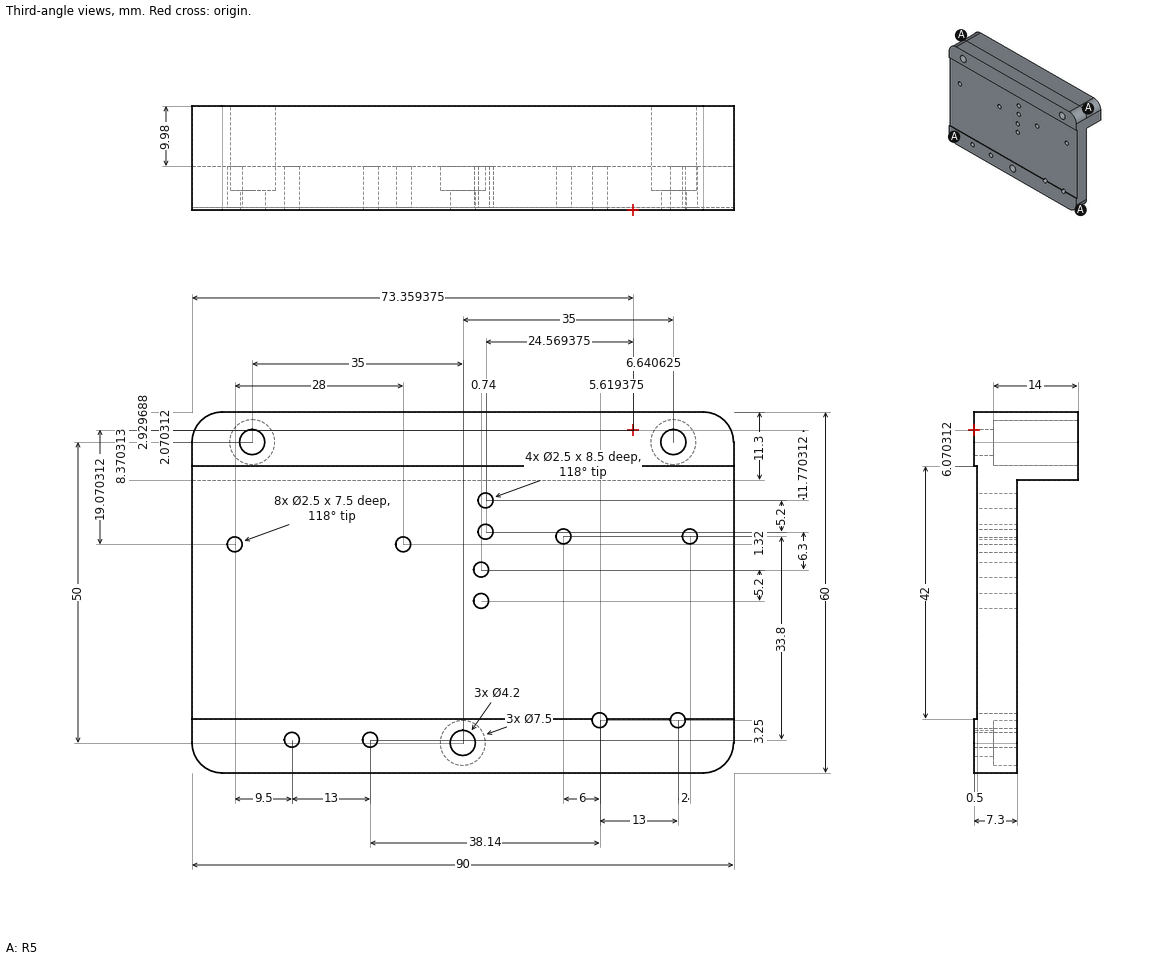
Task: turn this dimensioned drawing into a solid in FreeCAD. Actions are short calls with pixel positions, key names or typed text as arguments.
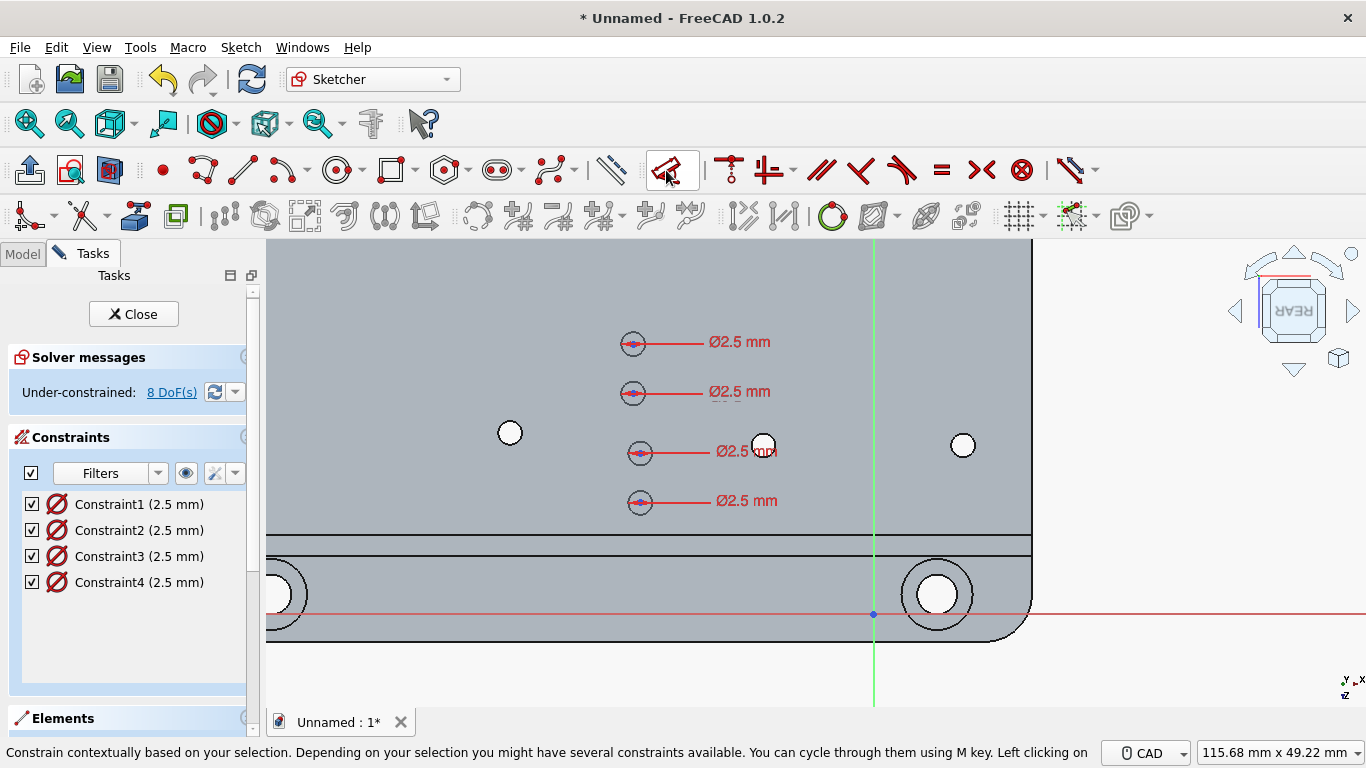
click(640, 503)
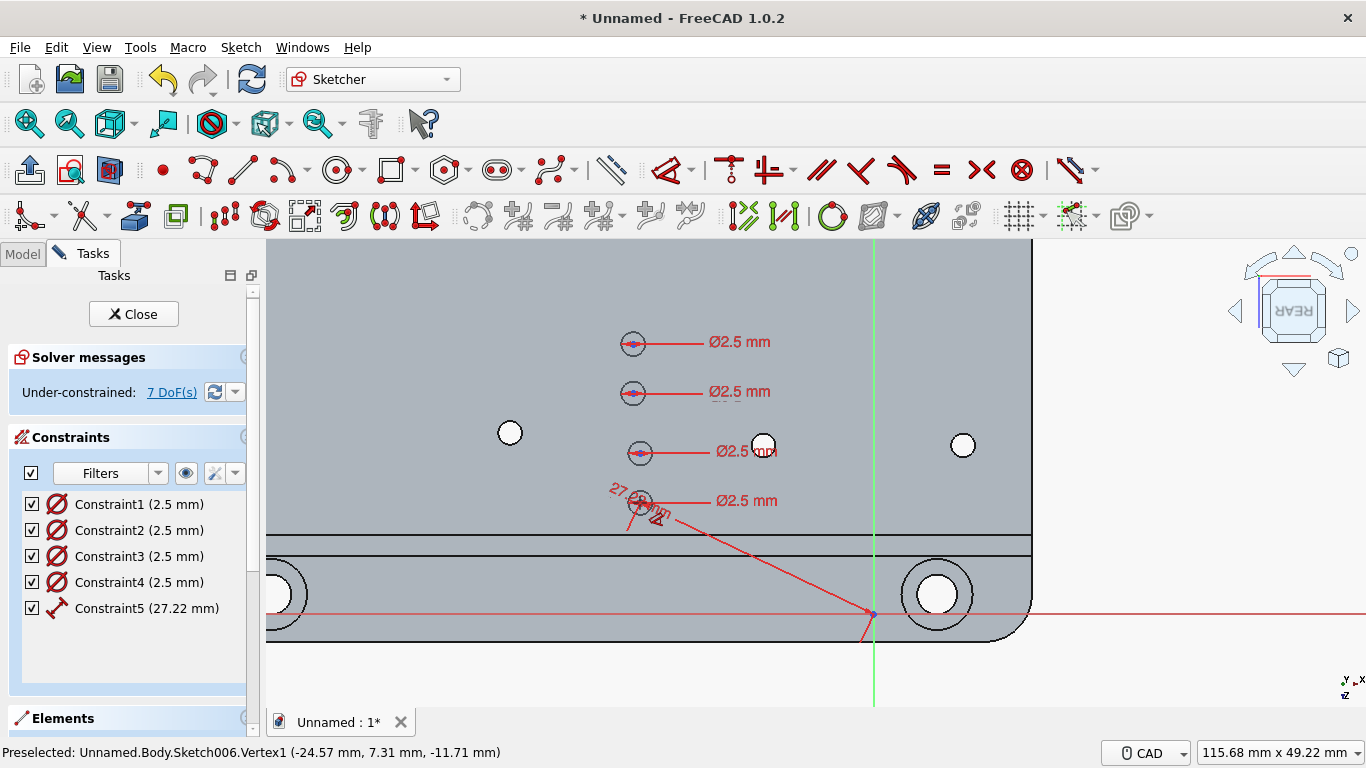
click(640, 453)
click(606, 478)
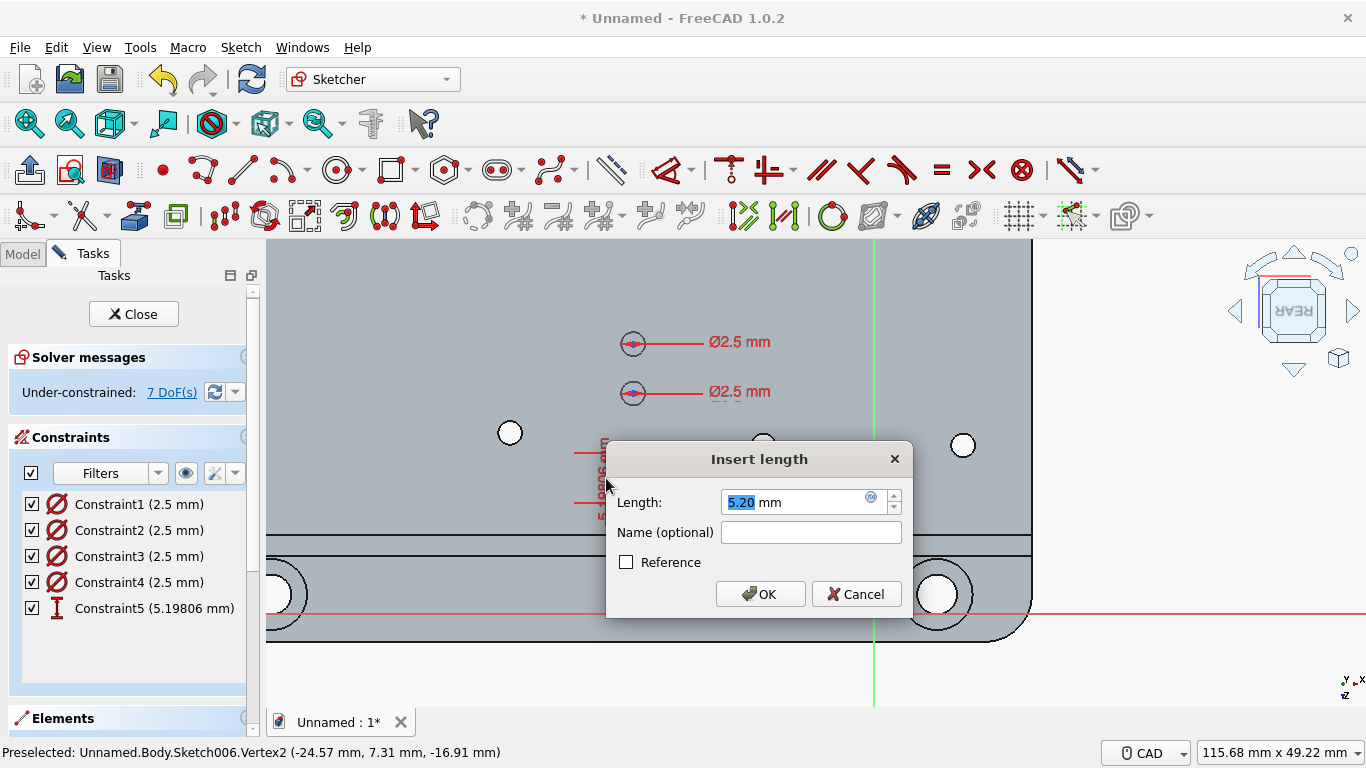
text(5.2)
key(Return)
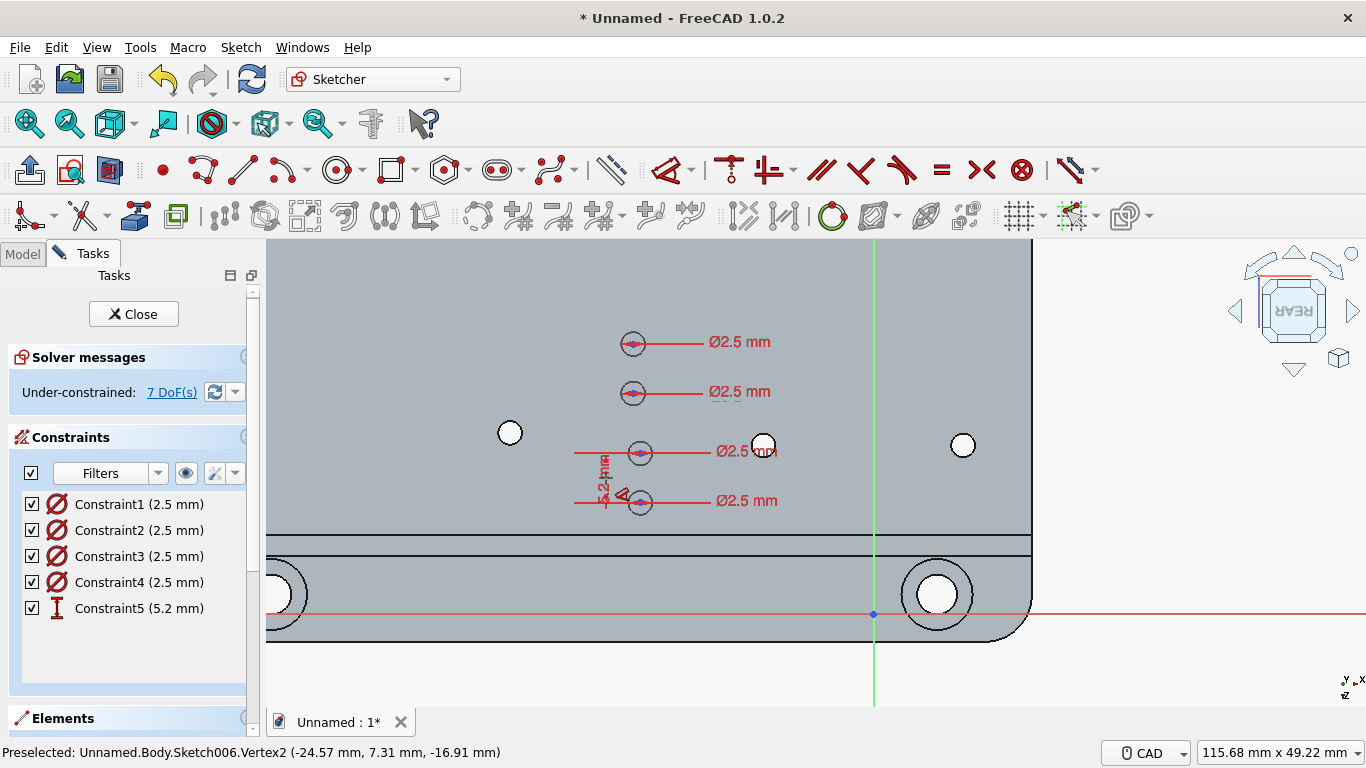
click(640, 453)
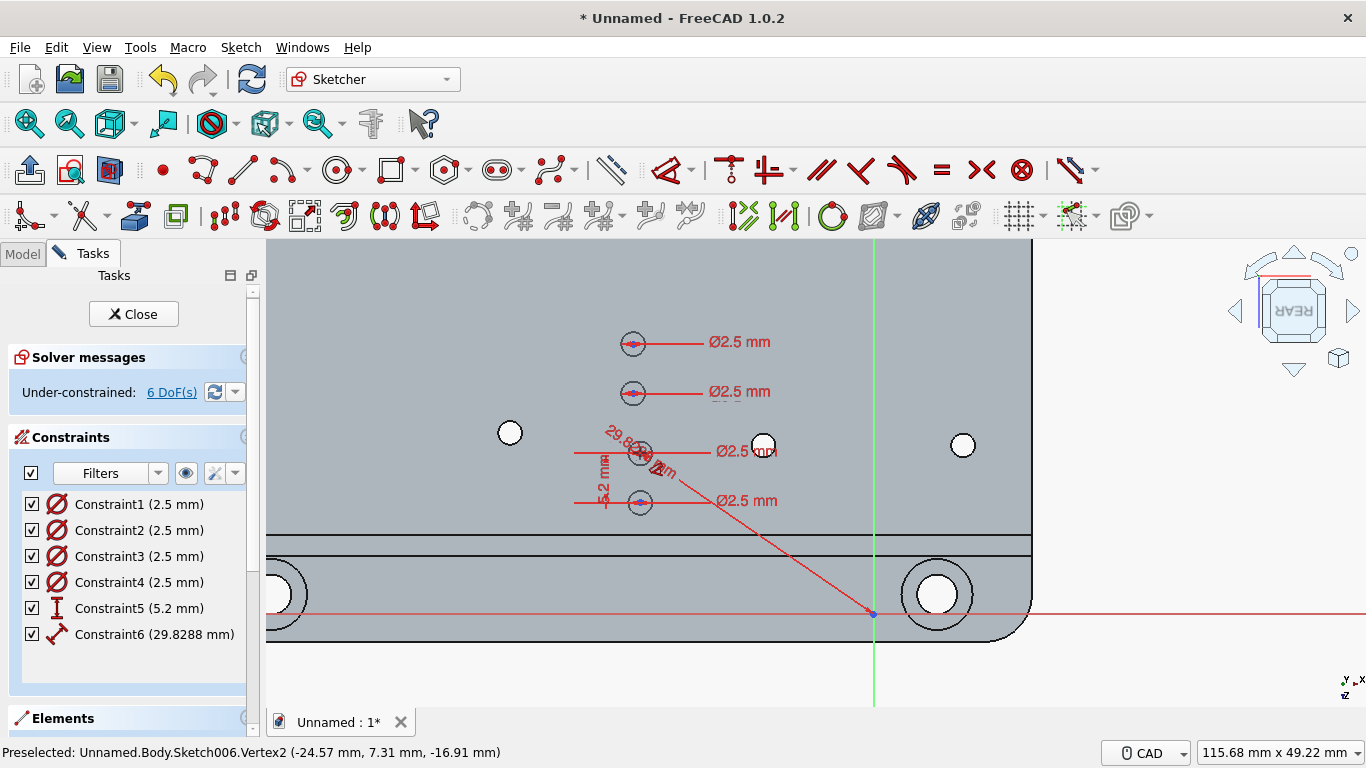
click(633, 394)
click(599, 423)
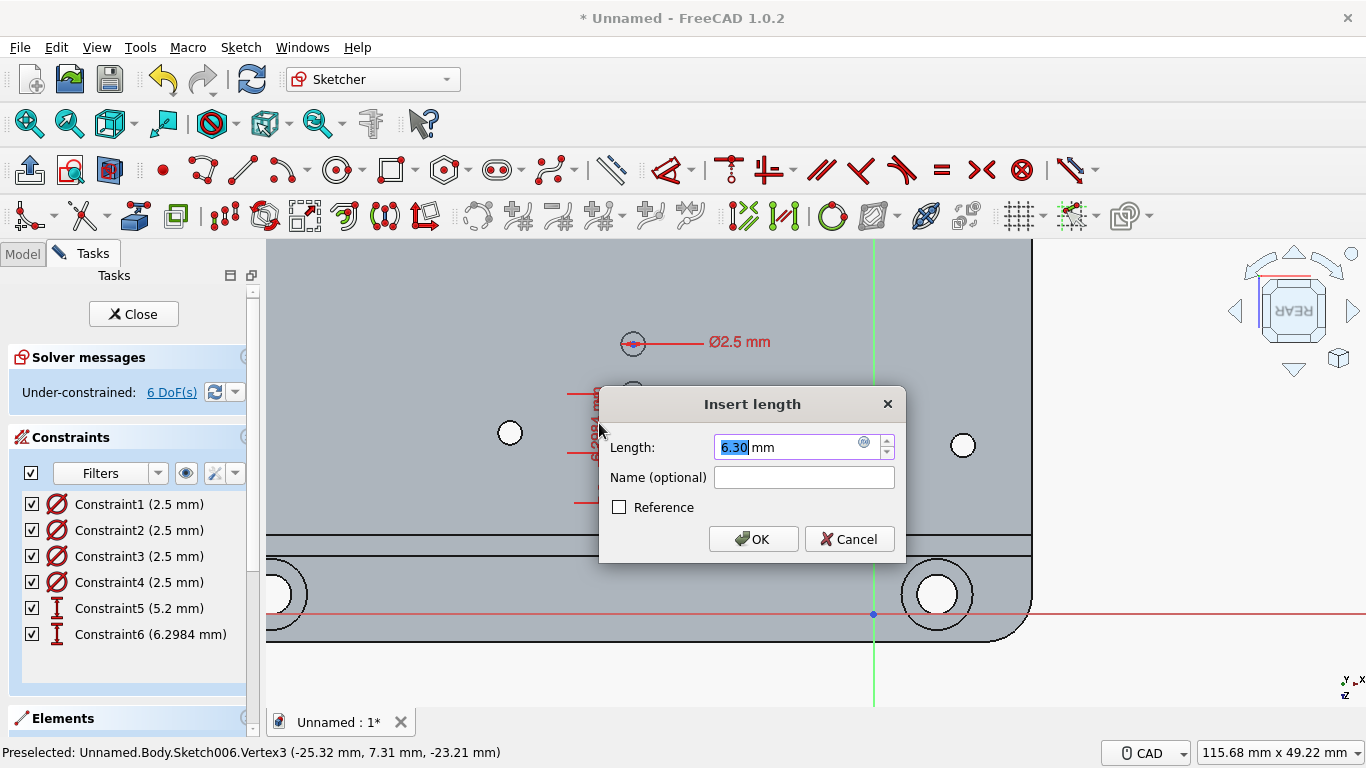
text(6.3)
key(Return)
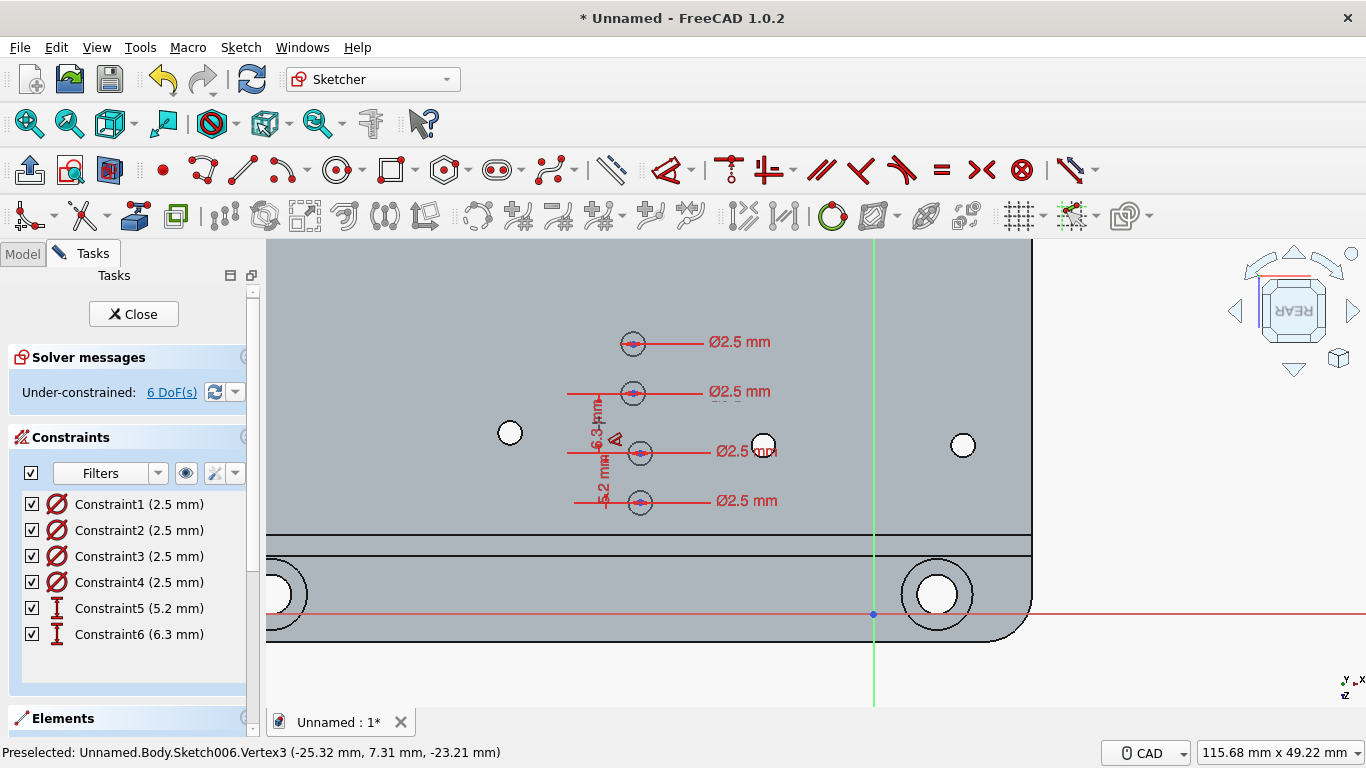
click(633, 394)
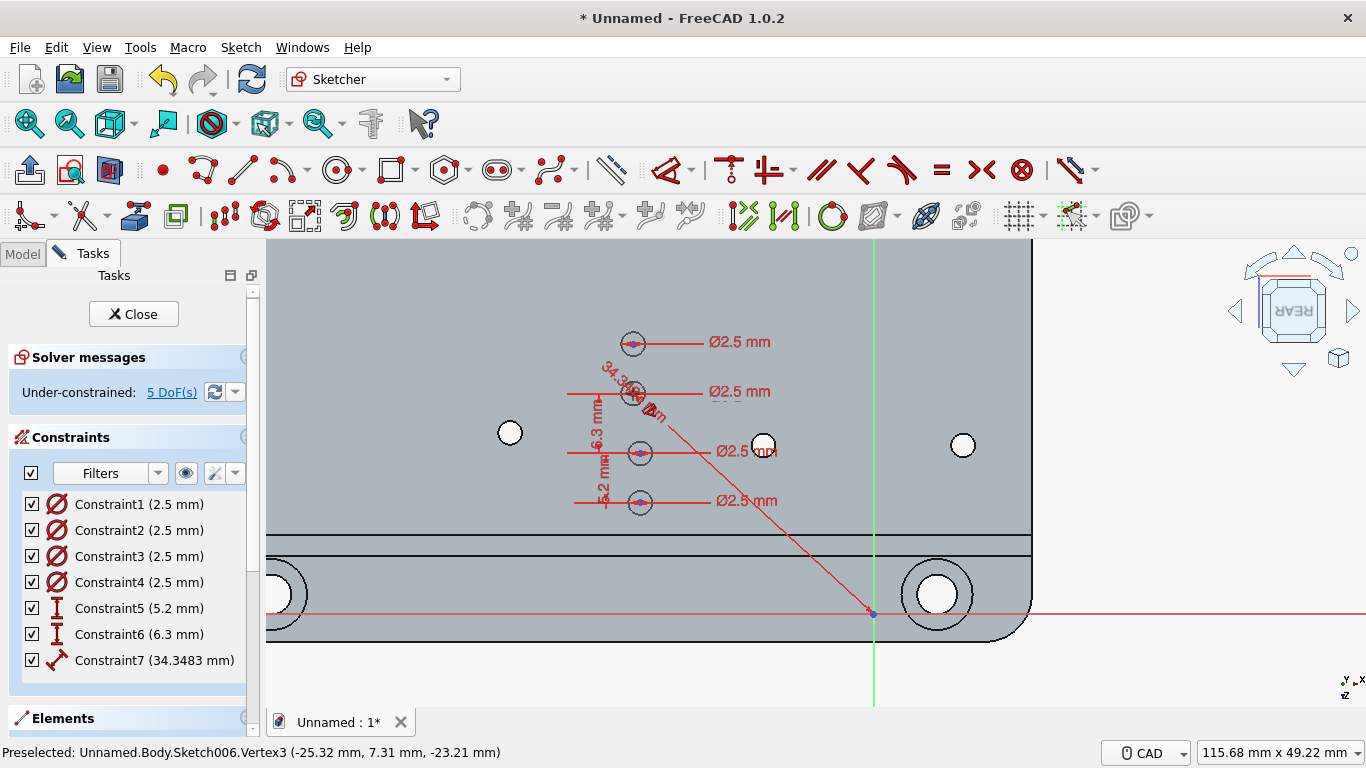
click(633, 344)
click(599, 369)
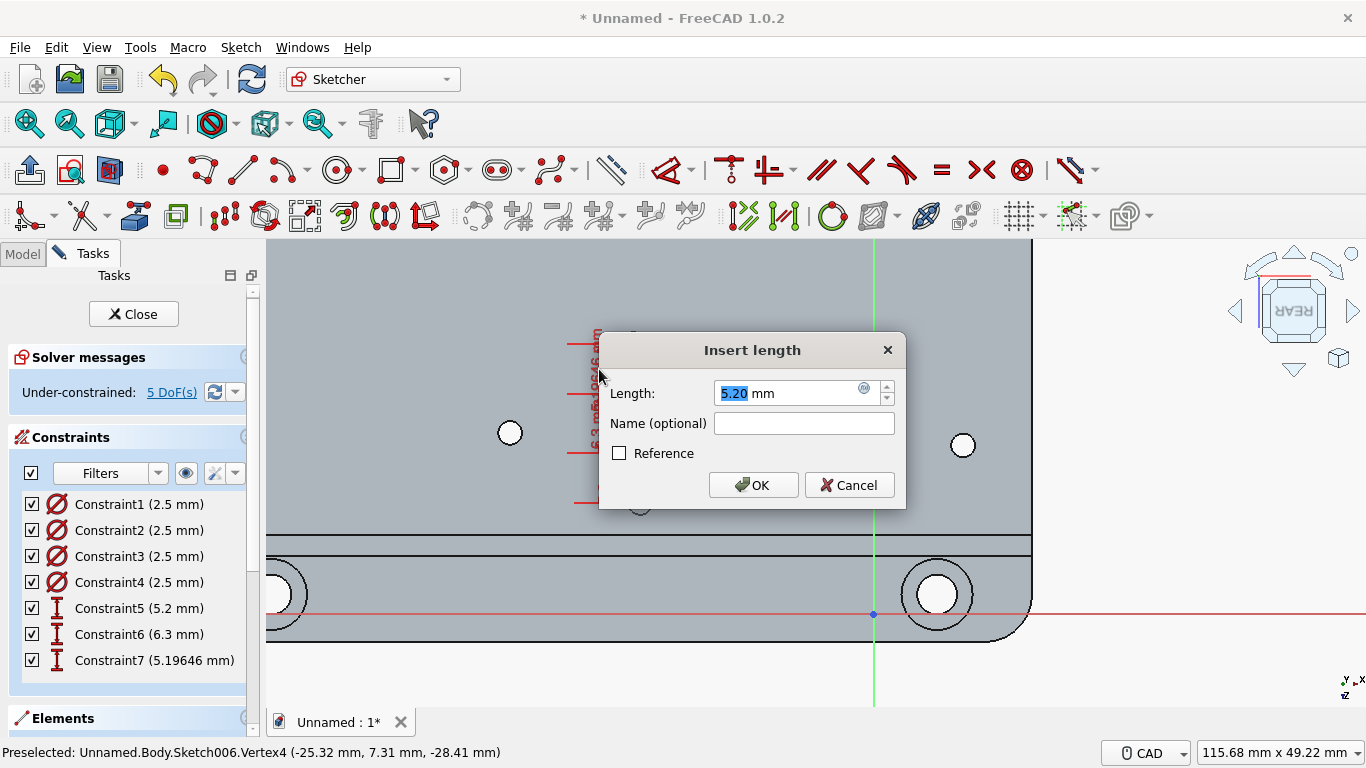
text(5.2)
key(Return)